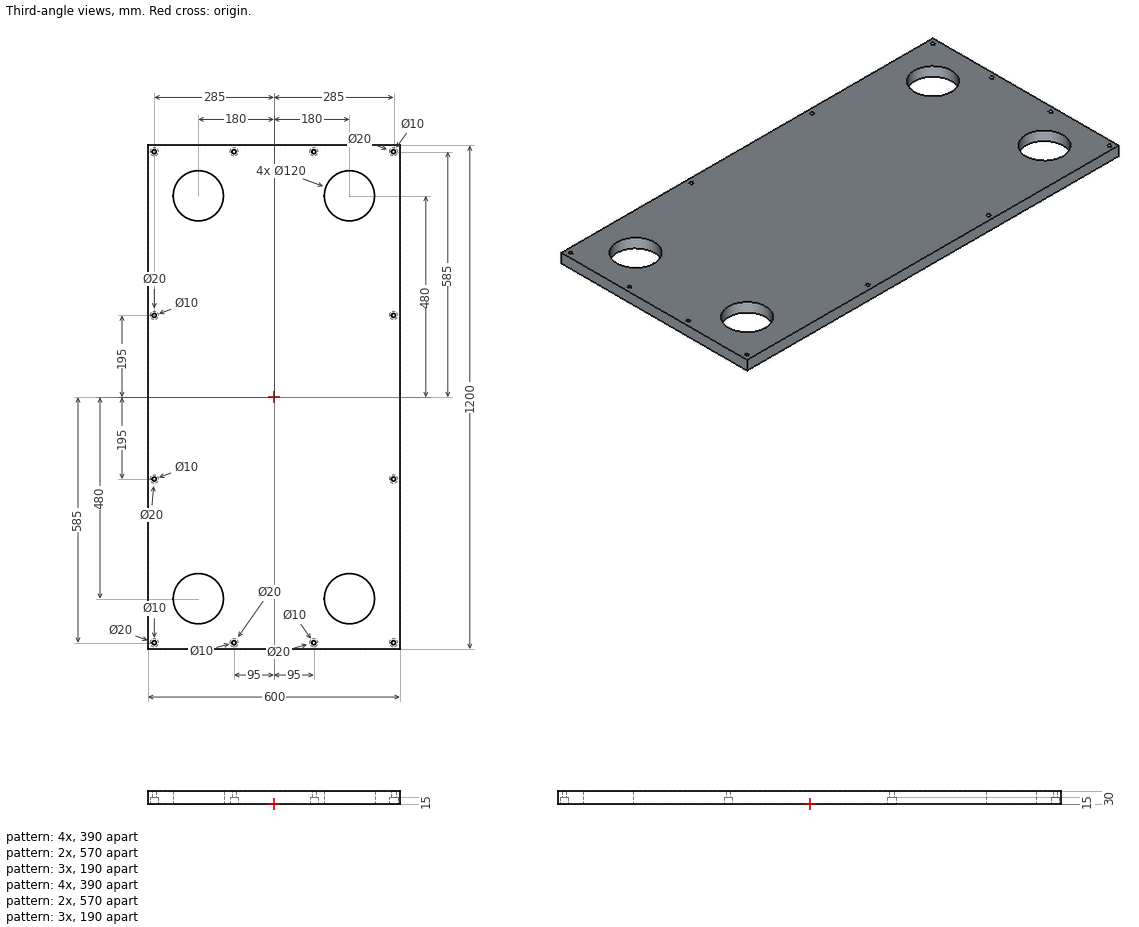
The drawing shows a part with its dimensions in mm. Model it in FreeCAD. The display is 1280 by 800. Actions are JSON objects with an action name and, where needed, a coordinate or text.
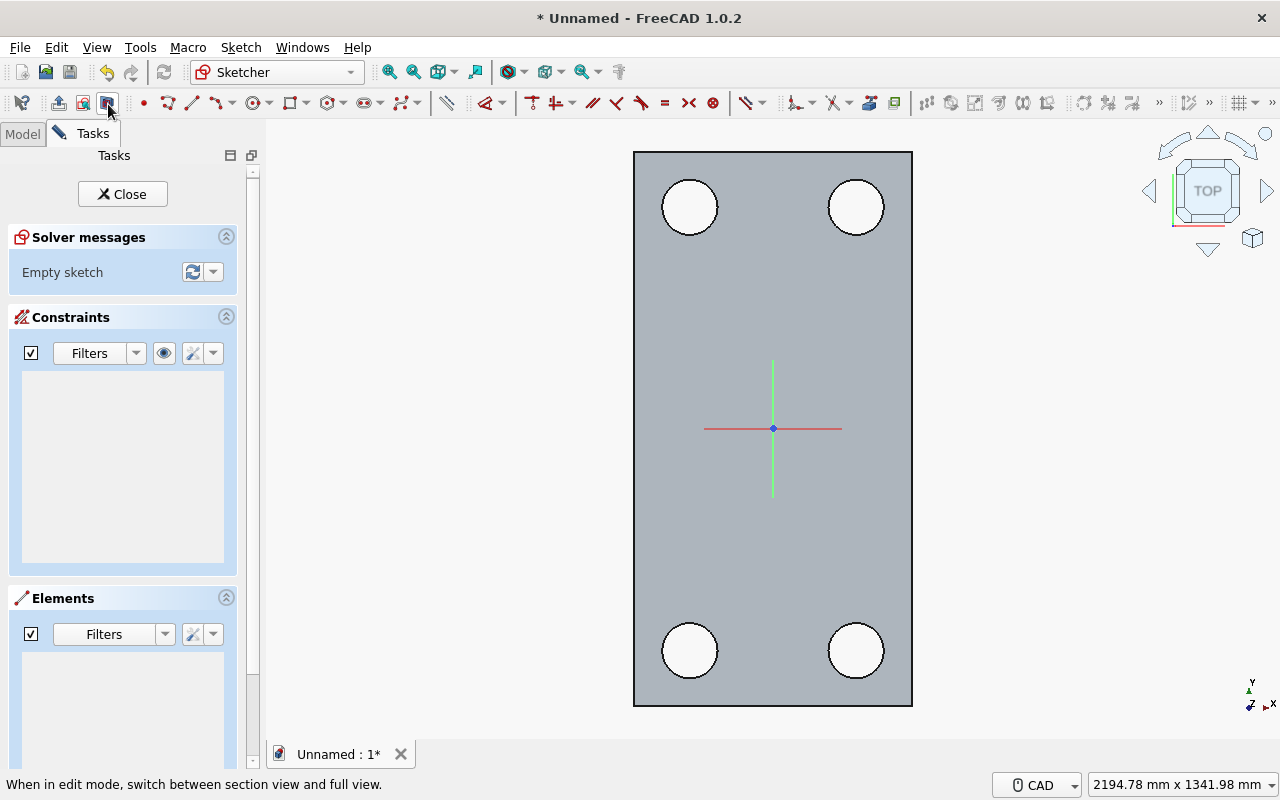
{"action": "scroll", "coordinate": [915, 147], "scroll_direction": "up", "scroll_amount": 15}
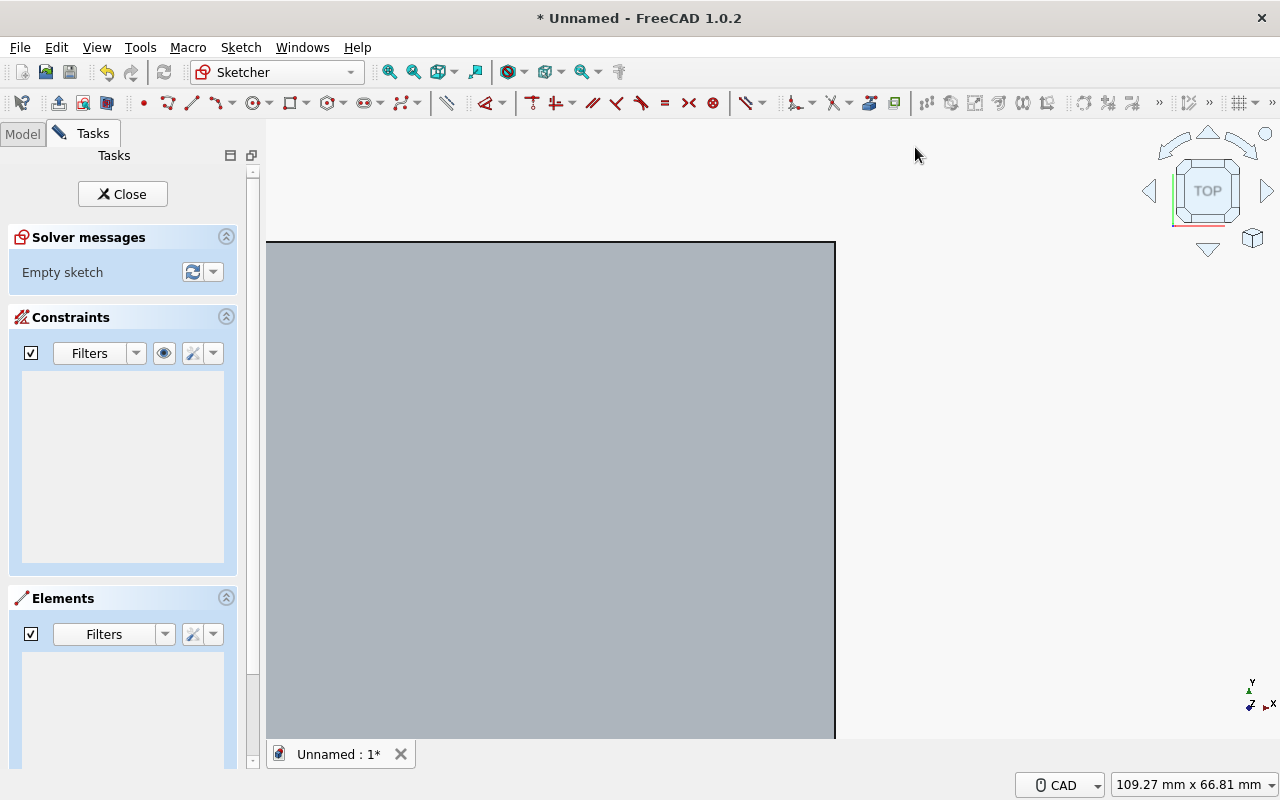
{"action": "scroll", "coordinate": [692, 366], "scroll_direction": "up", "scroll_amount": 7}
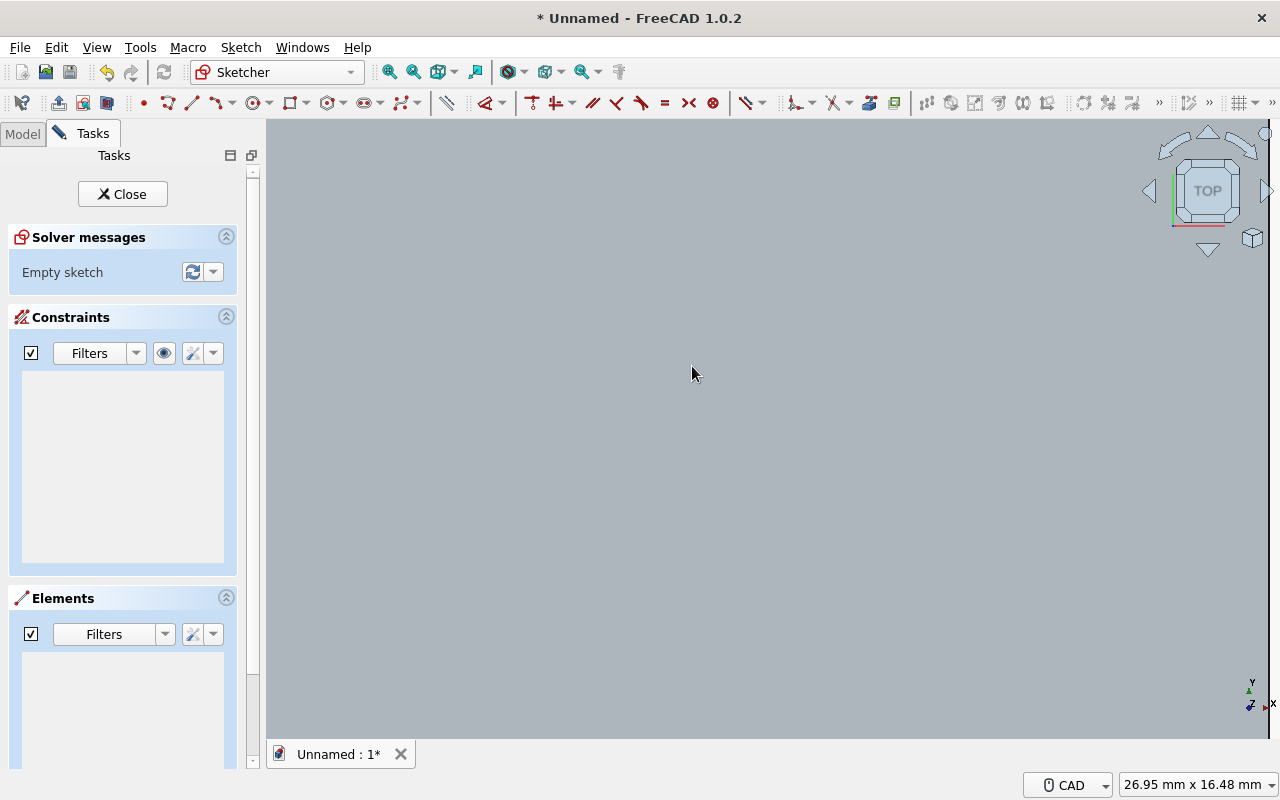
{"action": "key", "text": "g c"}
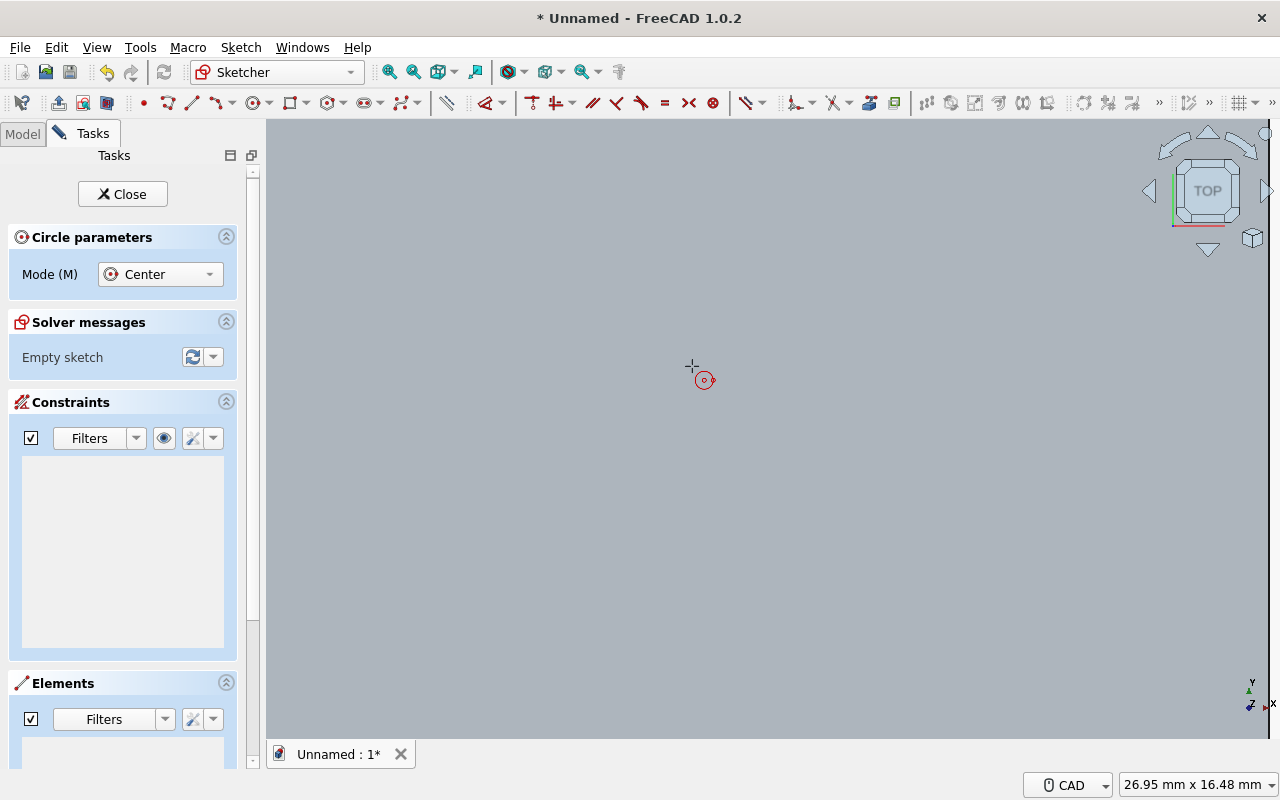
{"action": "left_click", "coordinate": [704, 428]}
{"action": "mouse_move", "coordinate": [837, 295]}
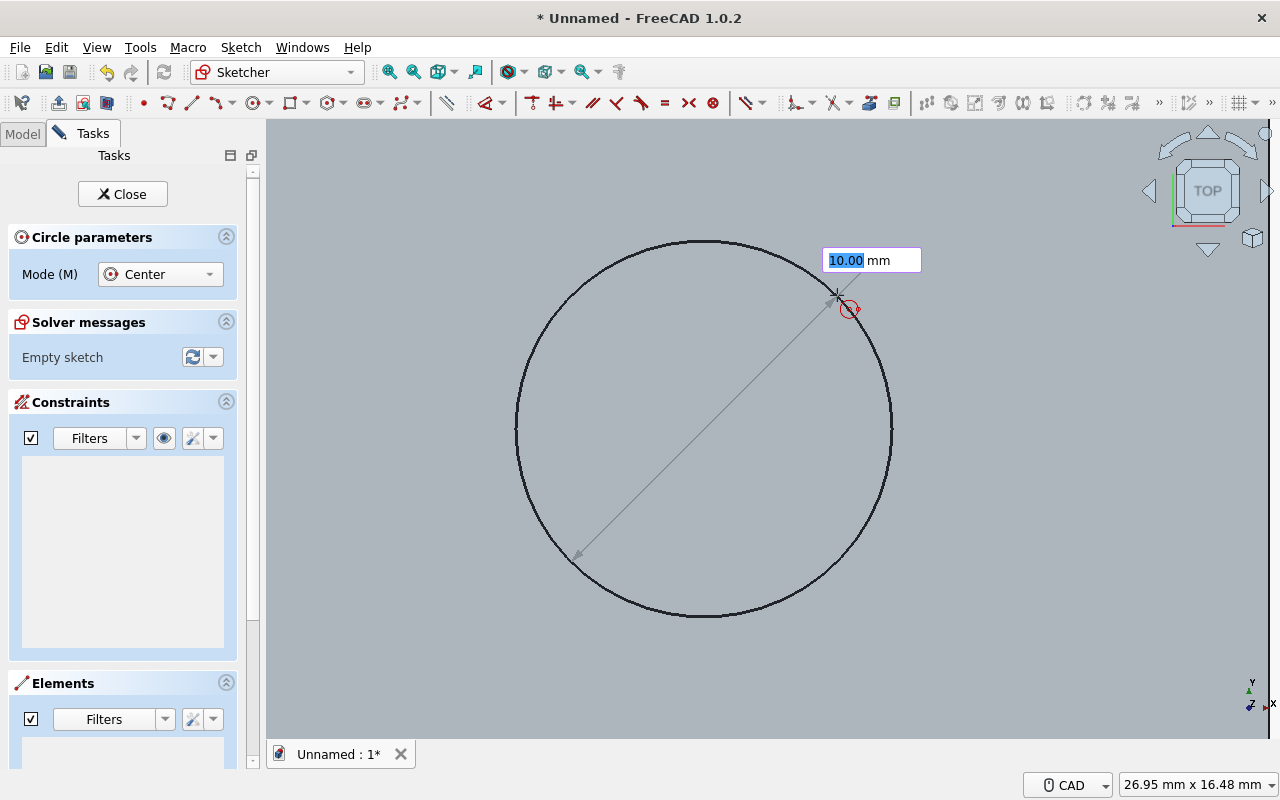
{"action": "type", "text": "10"}
{"action": "key", "text": "Return"}
{"action": "key", "text": "Escape"}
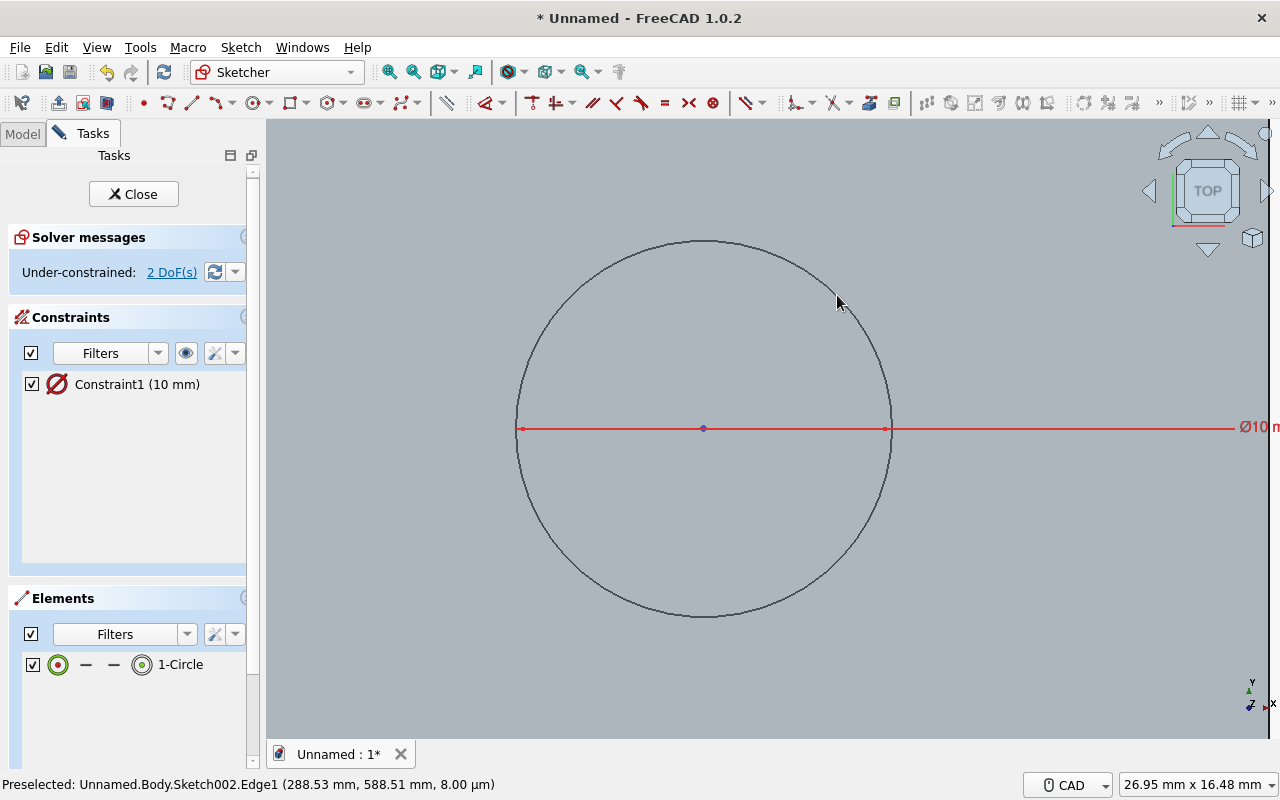
{"action": "left_click", "coordinate": [486, 104]}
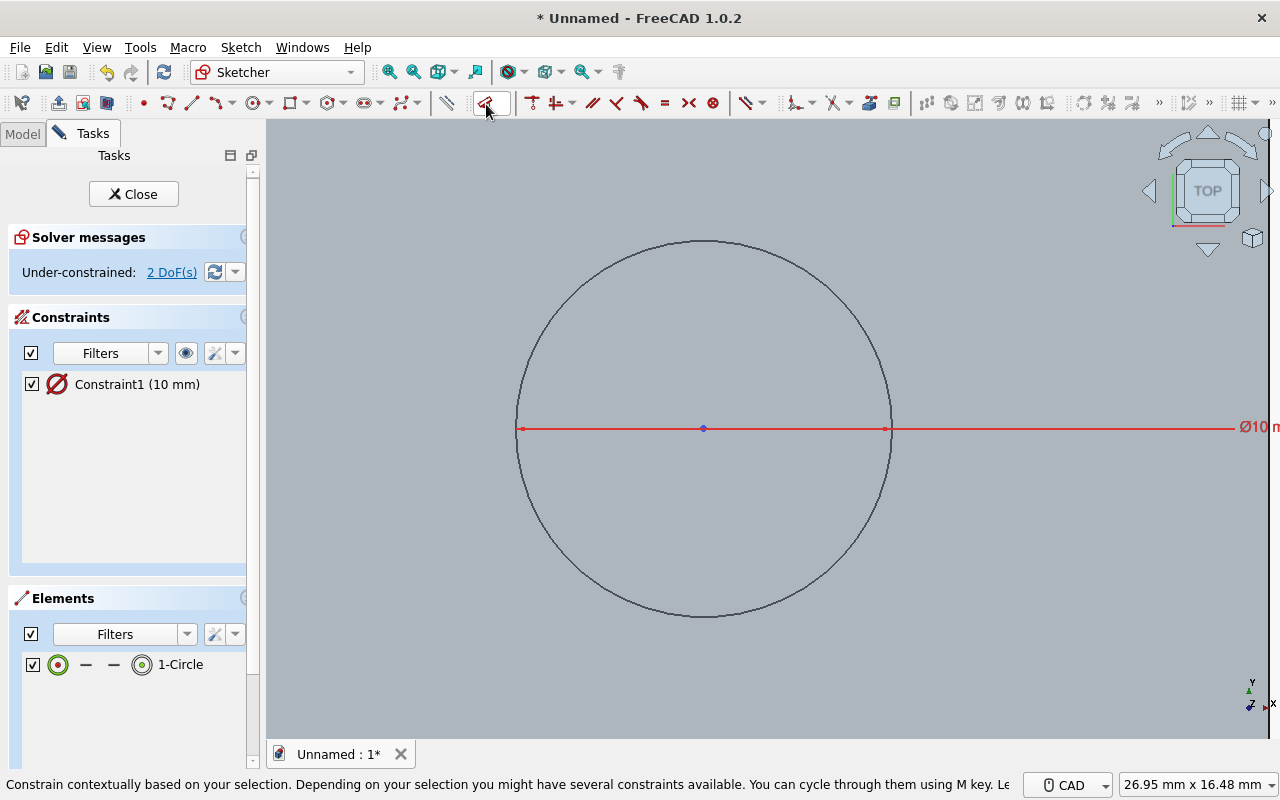
{"action": "left_click", "coordinate": [704, 429]}
{"action": "left_click", "coordinate": [499, 395]}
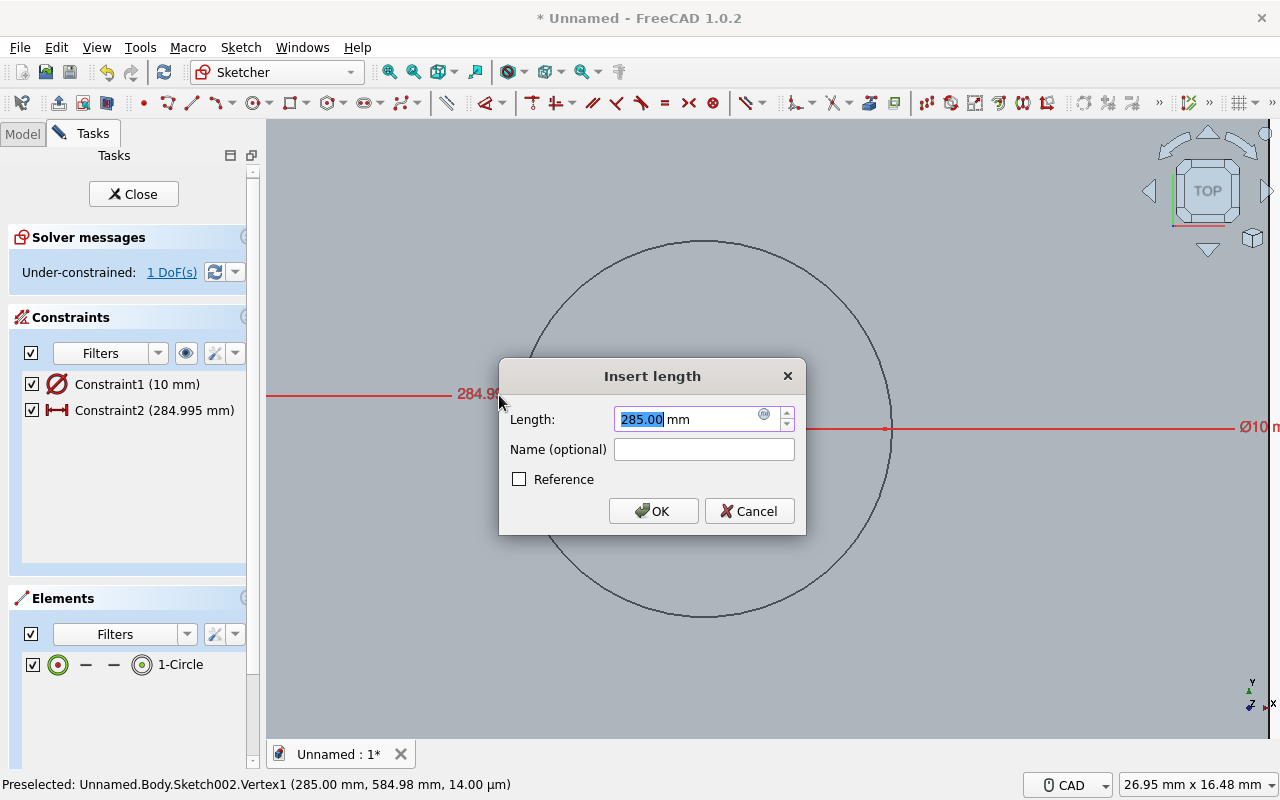
{"action": "type", "text": "285"}
{"action": "key", "text": "Return"}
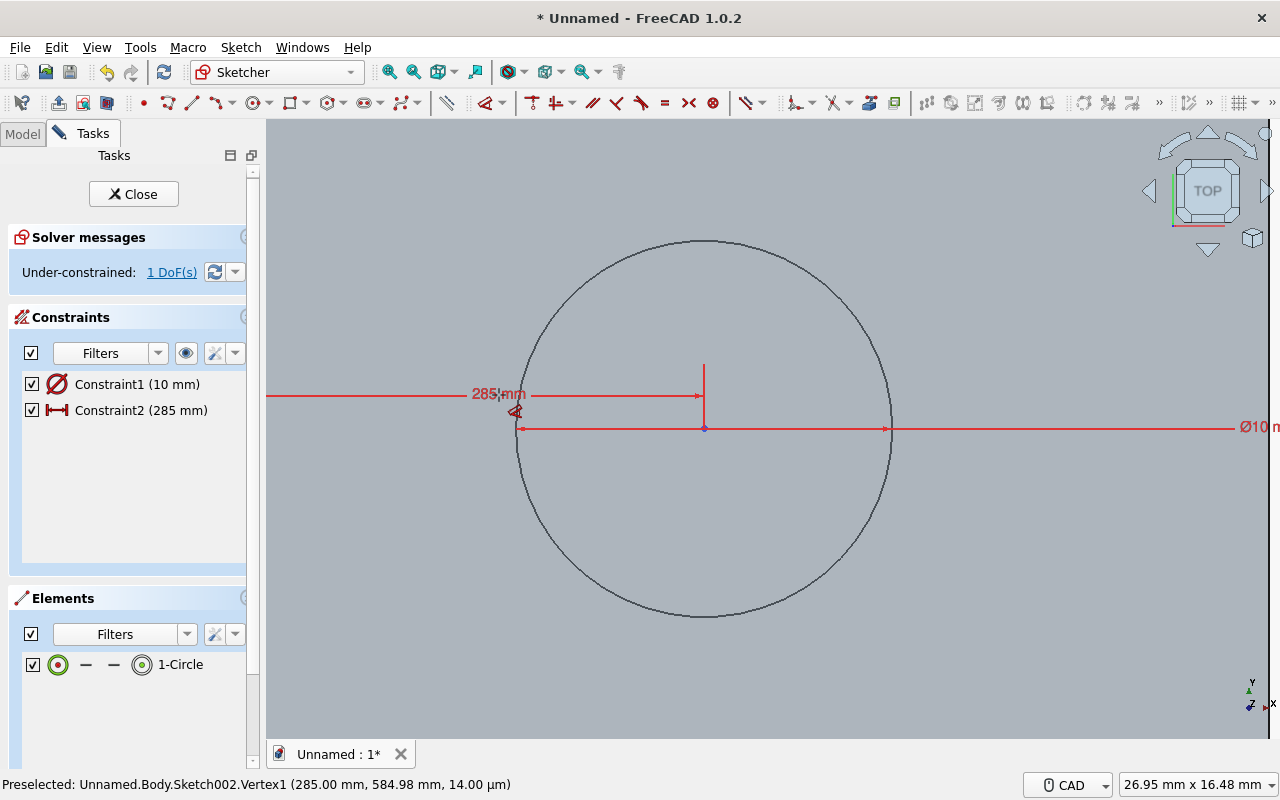
{"action": "left_click", "coordinate": [704, 429]}
{"action": "left_click", "coordinate": [738, 570]}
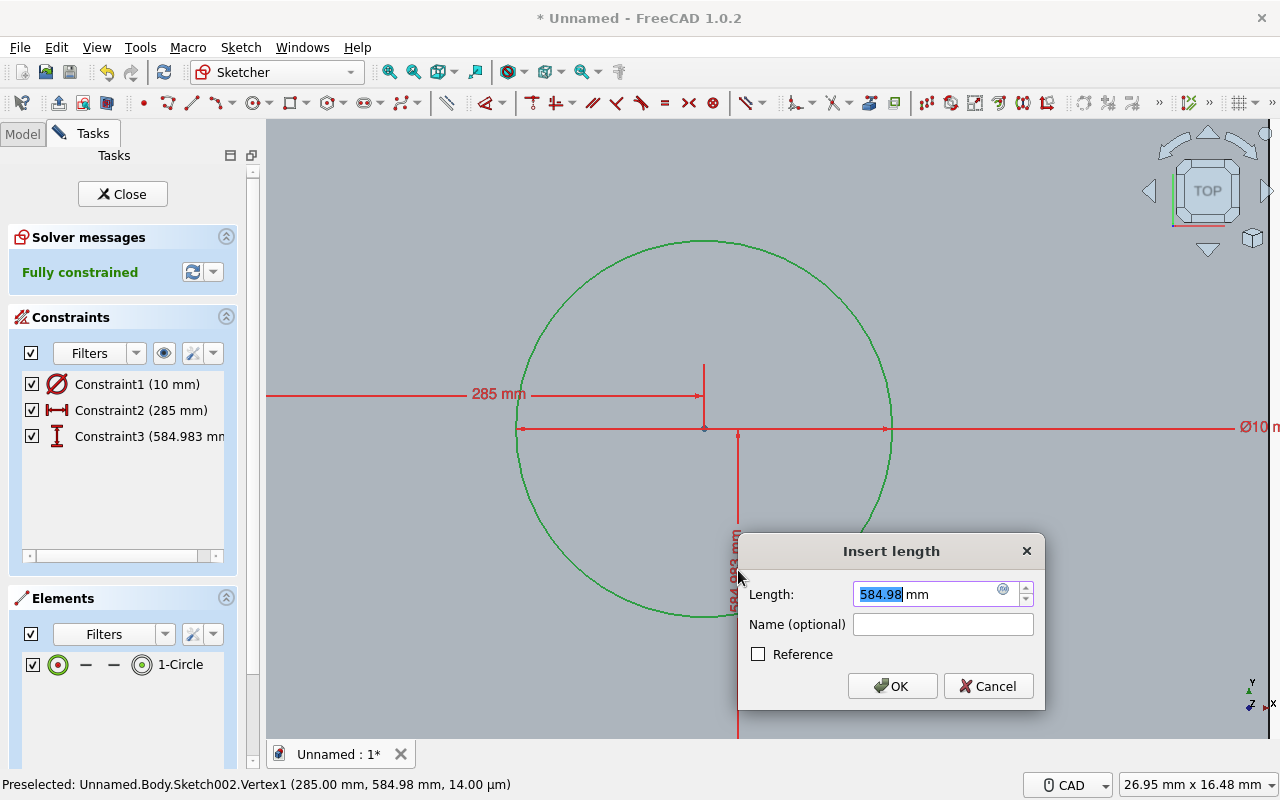
{"action": "type", "text": "585"}
{"action": "key", "text": "Return"}
{"action": "key", "text": "Escape"}